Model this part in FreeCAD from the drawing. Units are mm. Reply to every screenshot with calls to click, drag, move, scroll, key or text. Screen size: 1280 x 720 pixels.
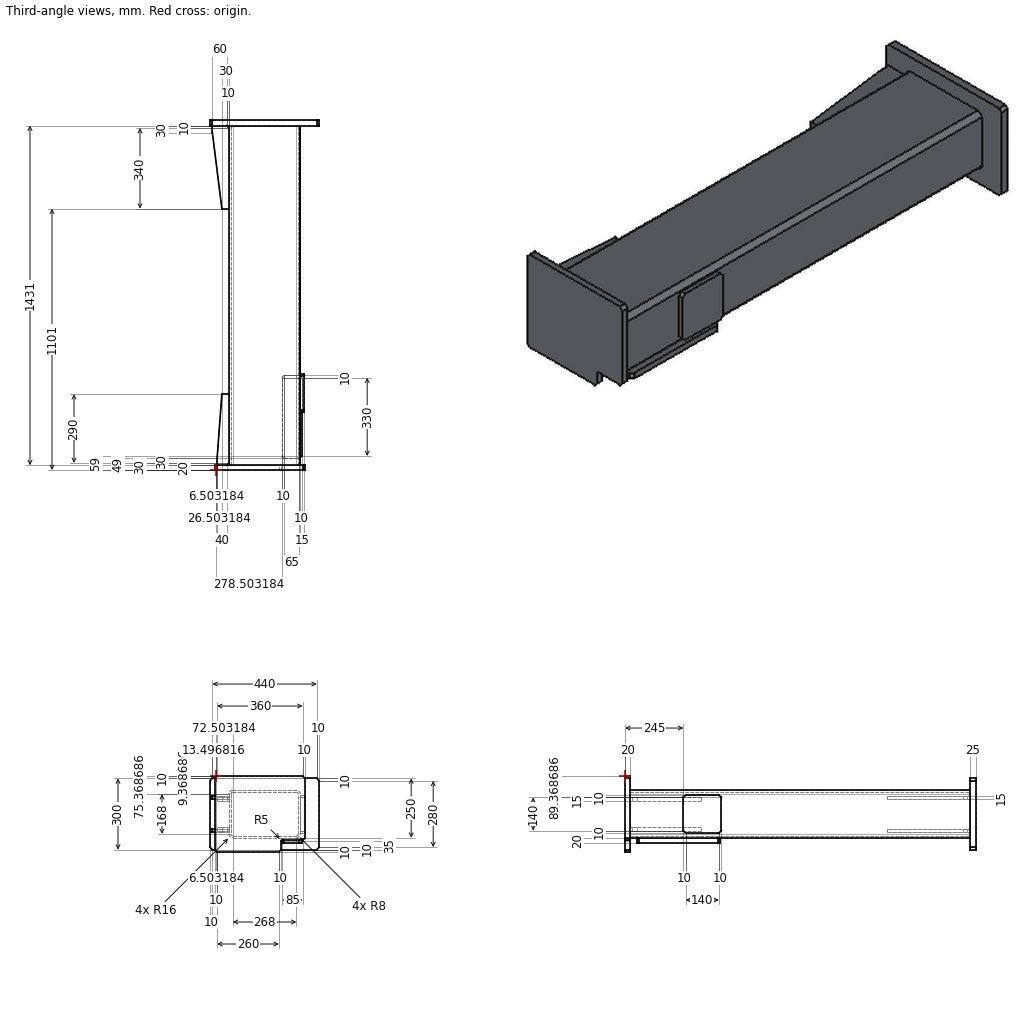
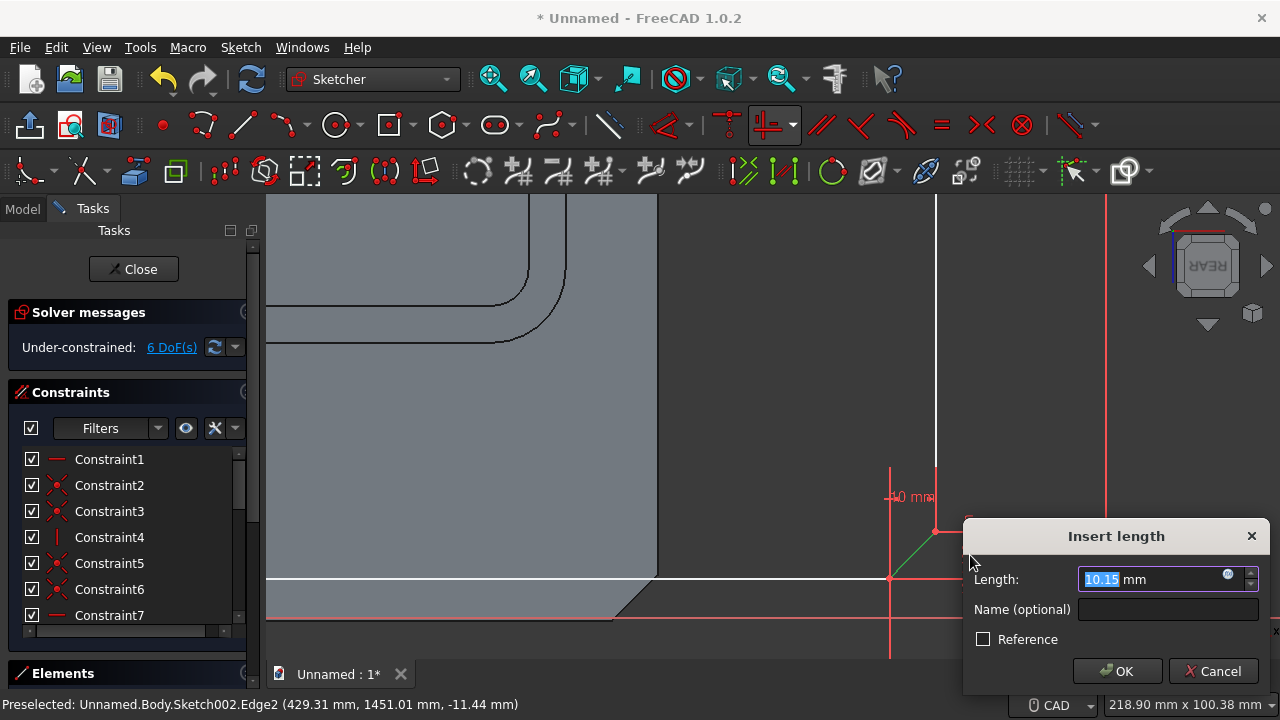
text(10)
key(Return)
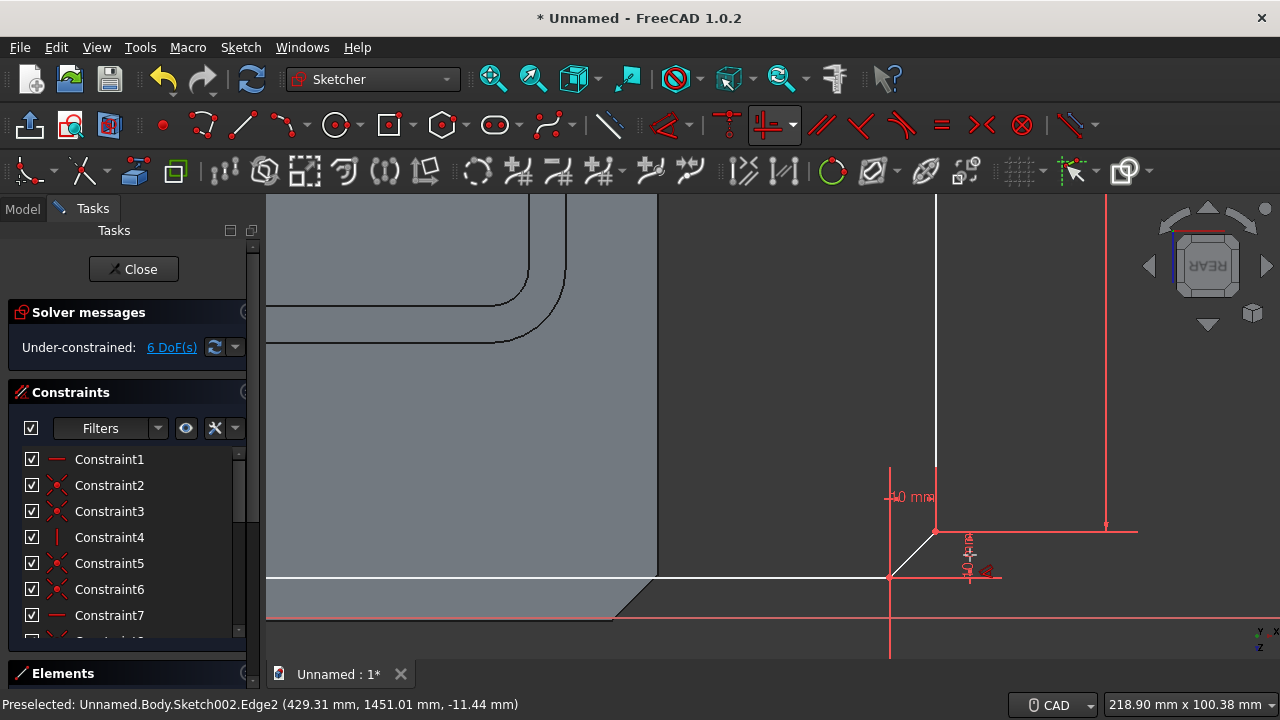
scroll(915, 559, down, 8)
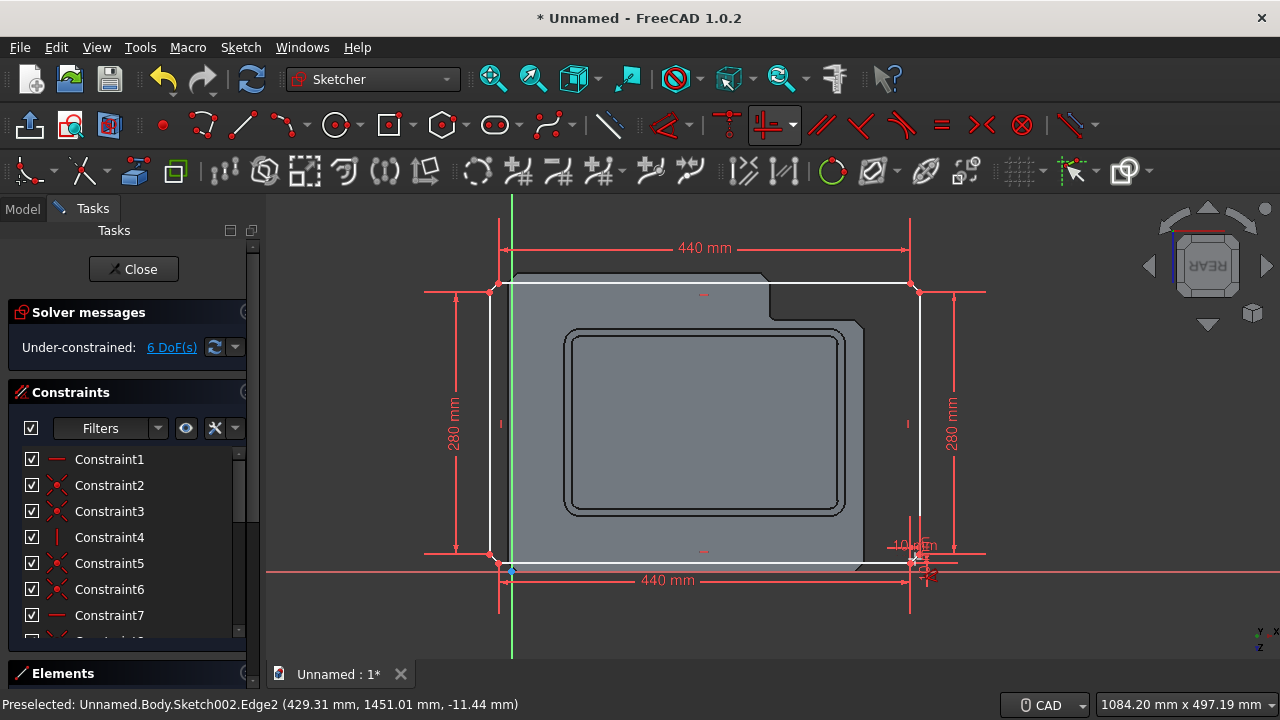
scroll(917, 289, up, 8)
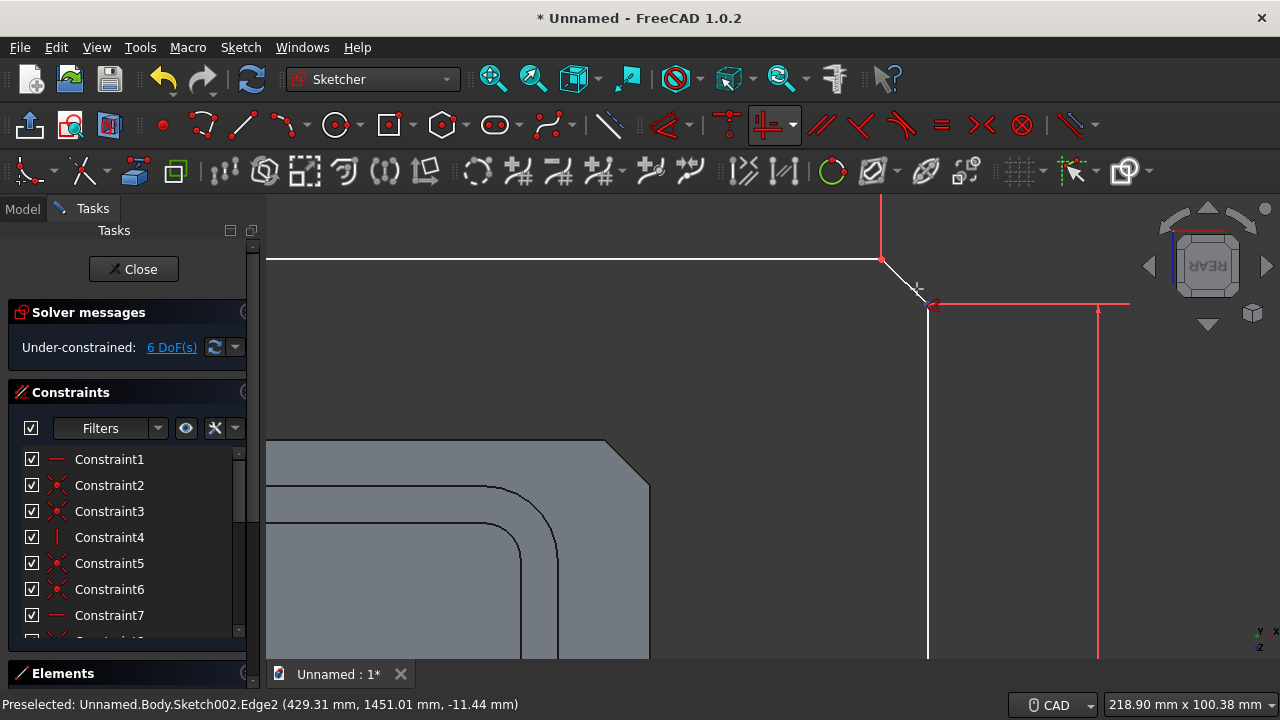
click(914, 291)
click(905, 225)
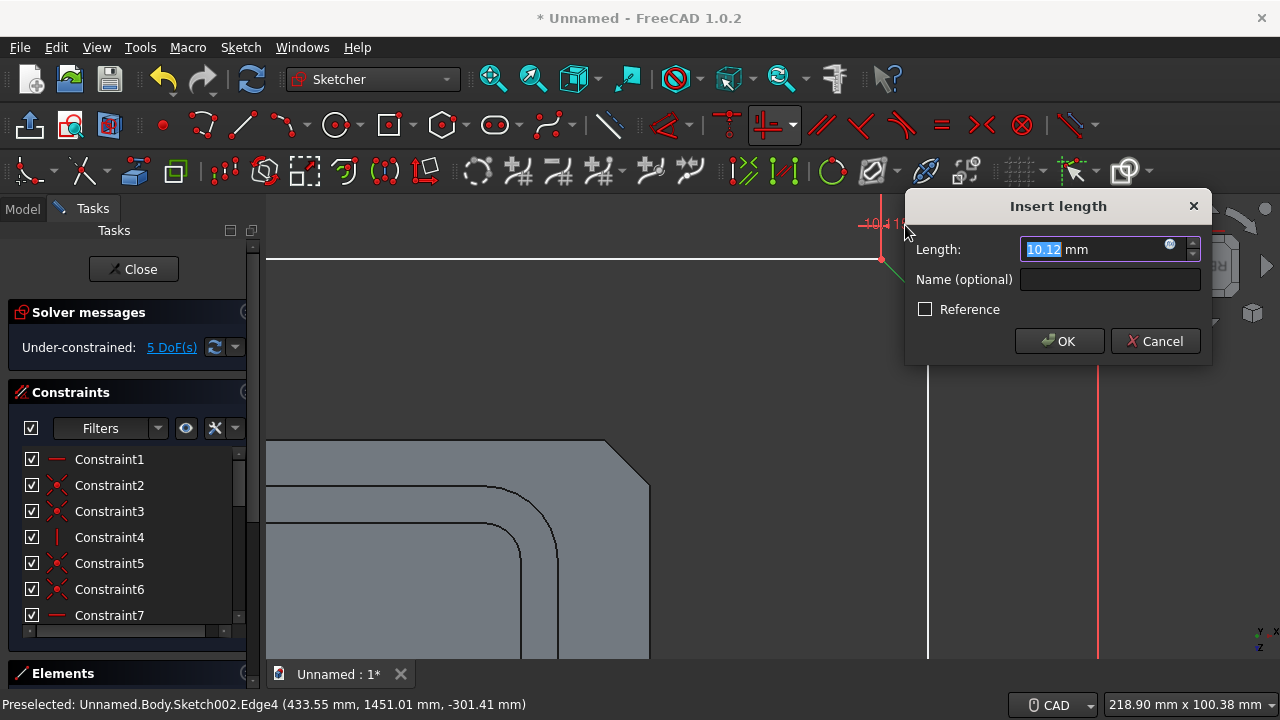
text(10)
key(Return)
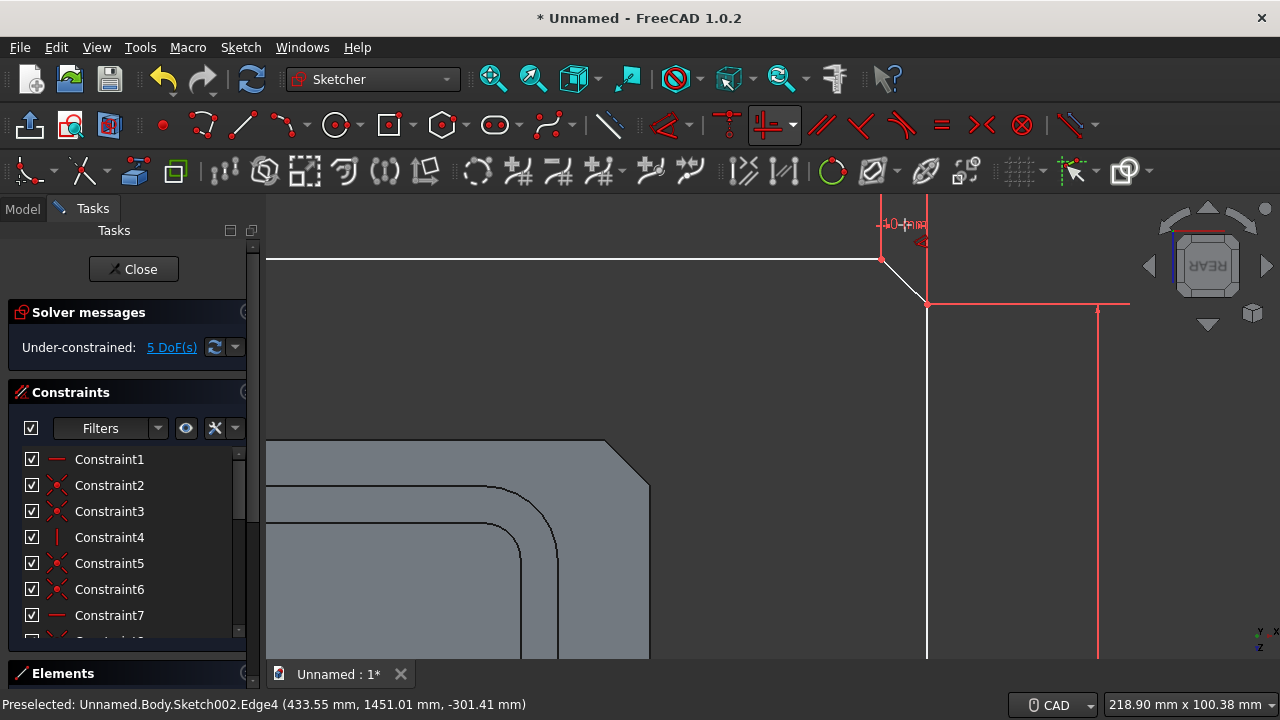
click(914, 291)
click(961, 282)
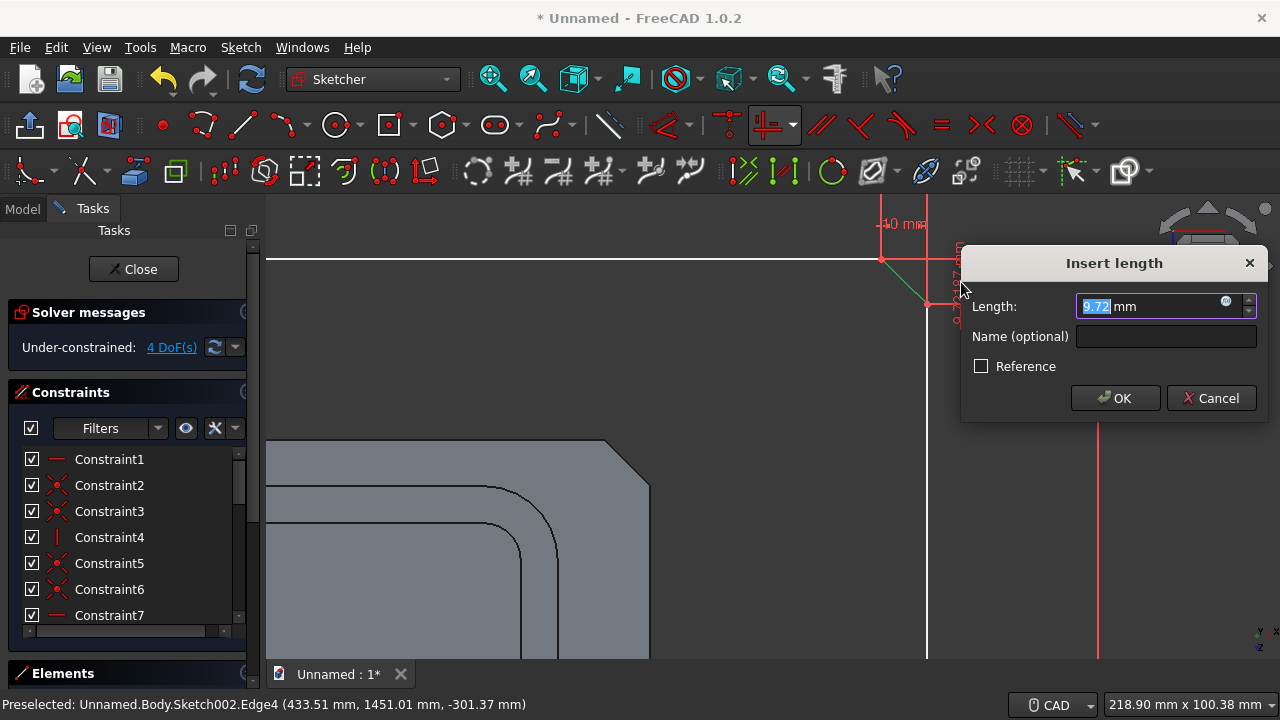
text(10)
key(Return)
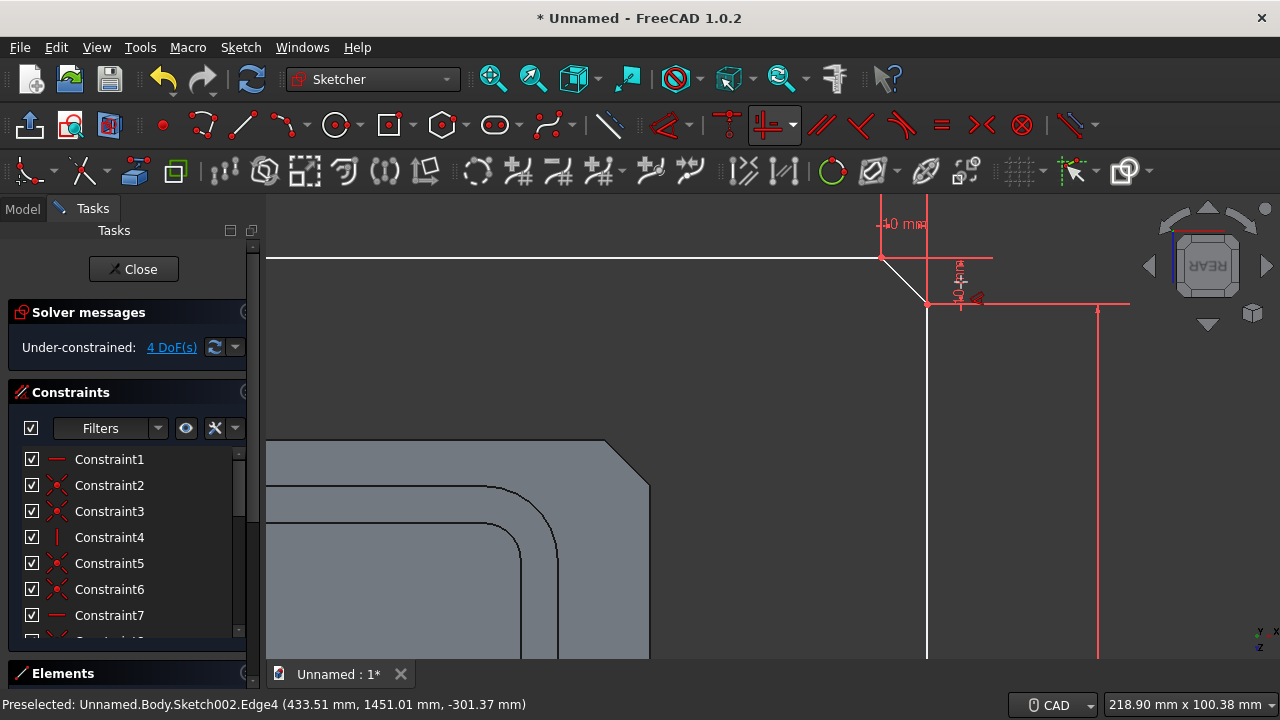
scroll(917, 289, down, 8)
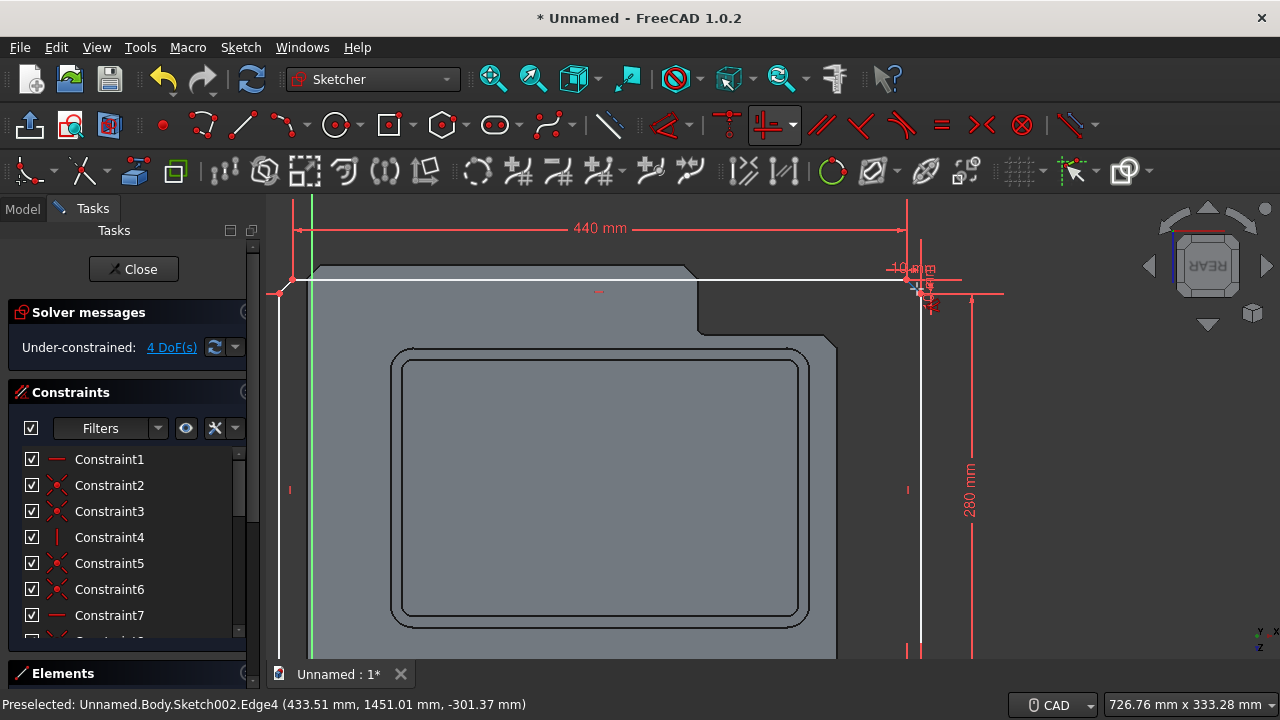
scroll(496, 286, up, 8)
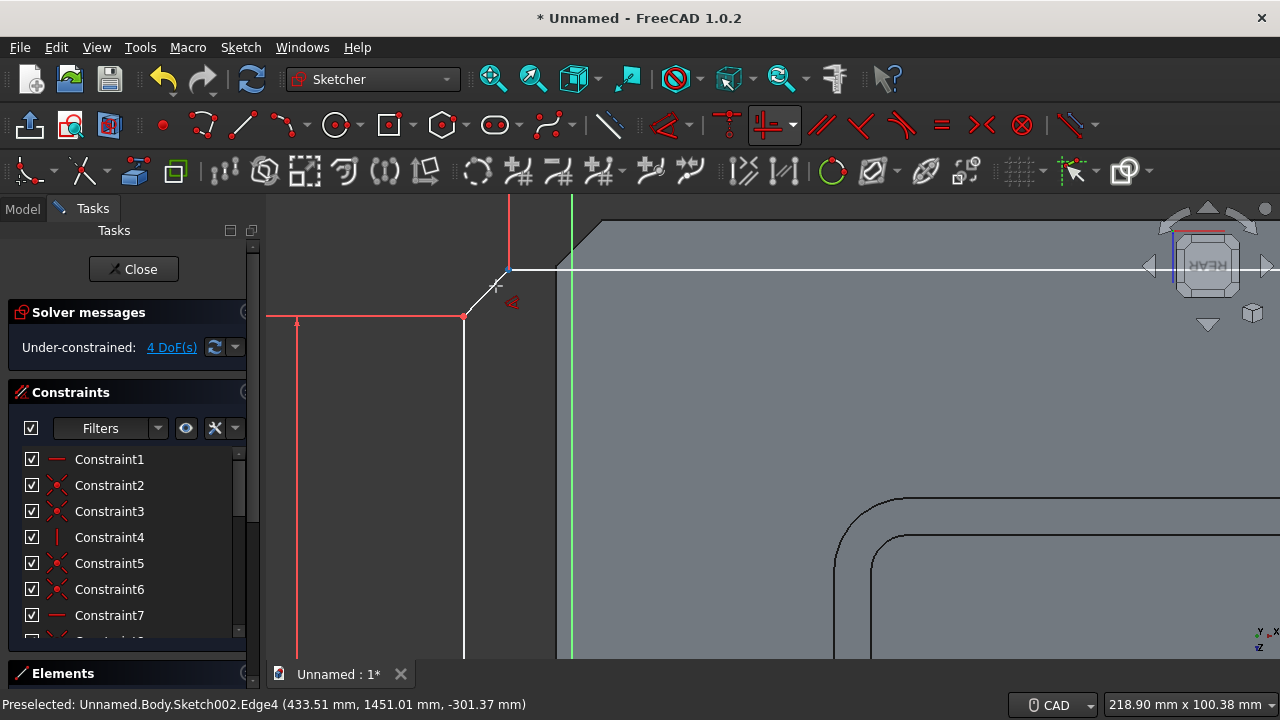
click(495, 284)
click(486, 236)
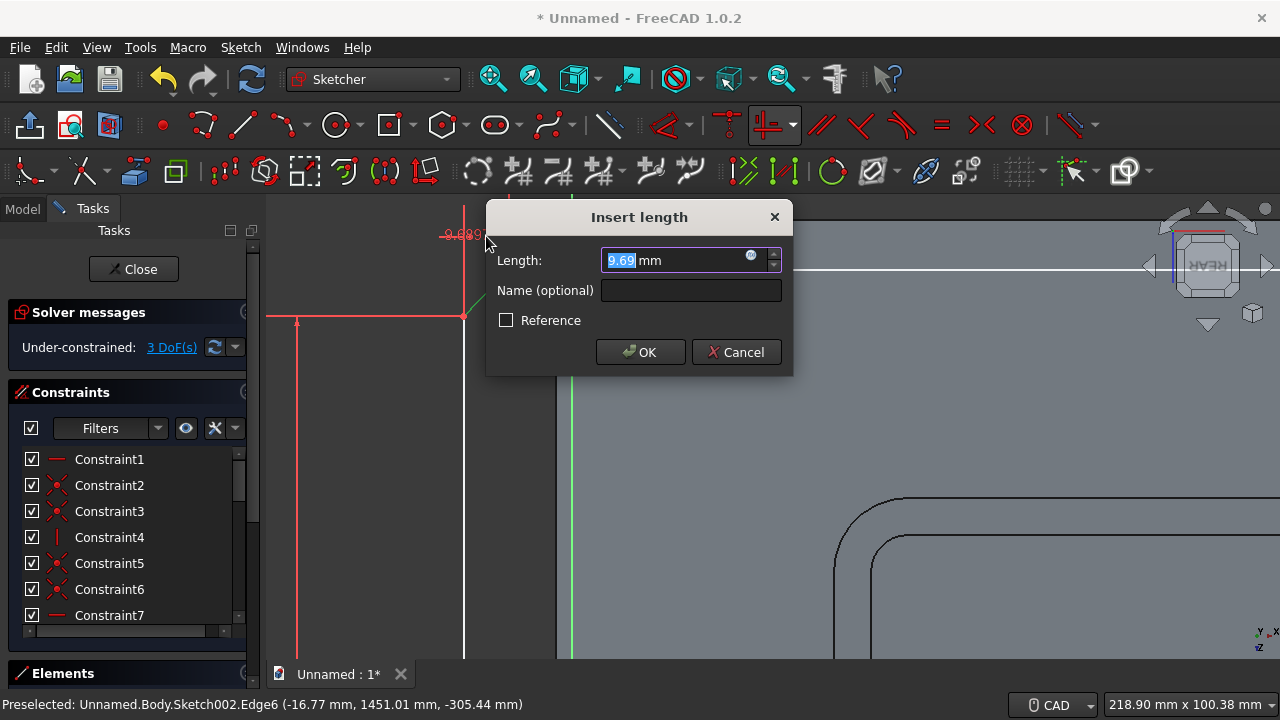
text(10)
key(Return)